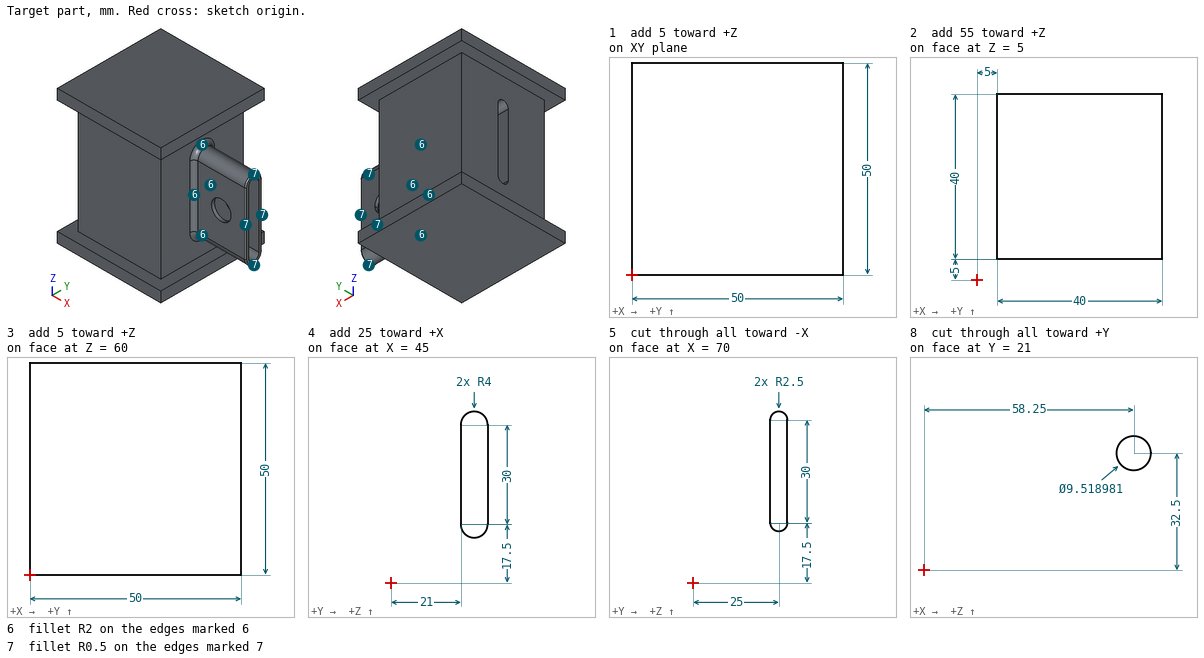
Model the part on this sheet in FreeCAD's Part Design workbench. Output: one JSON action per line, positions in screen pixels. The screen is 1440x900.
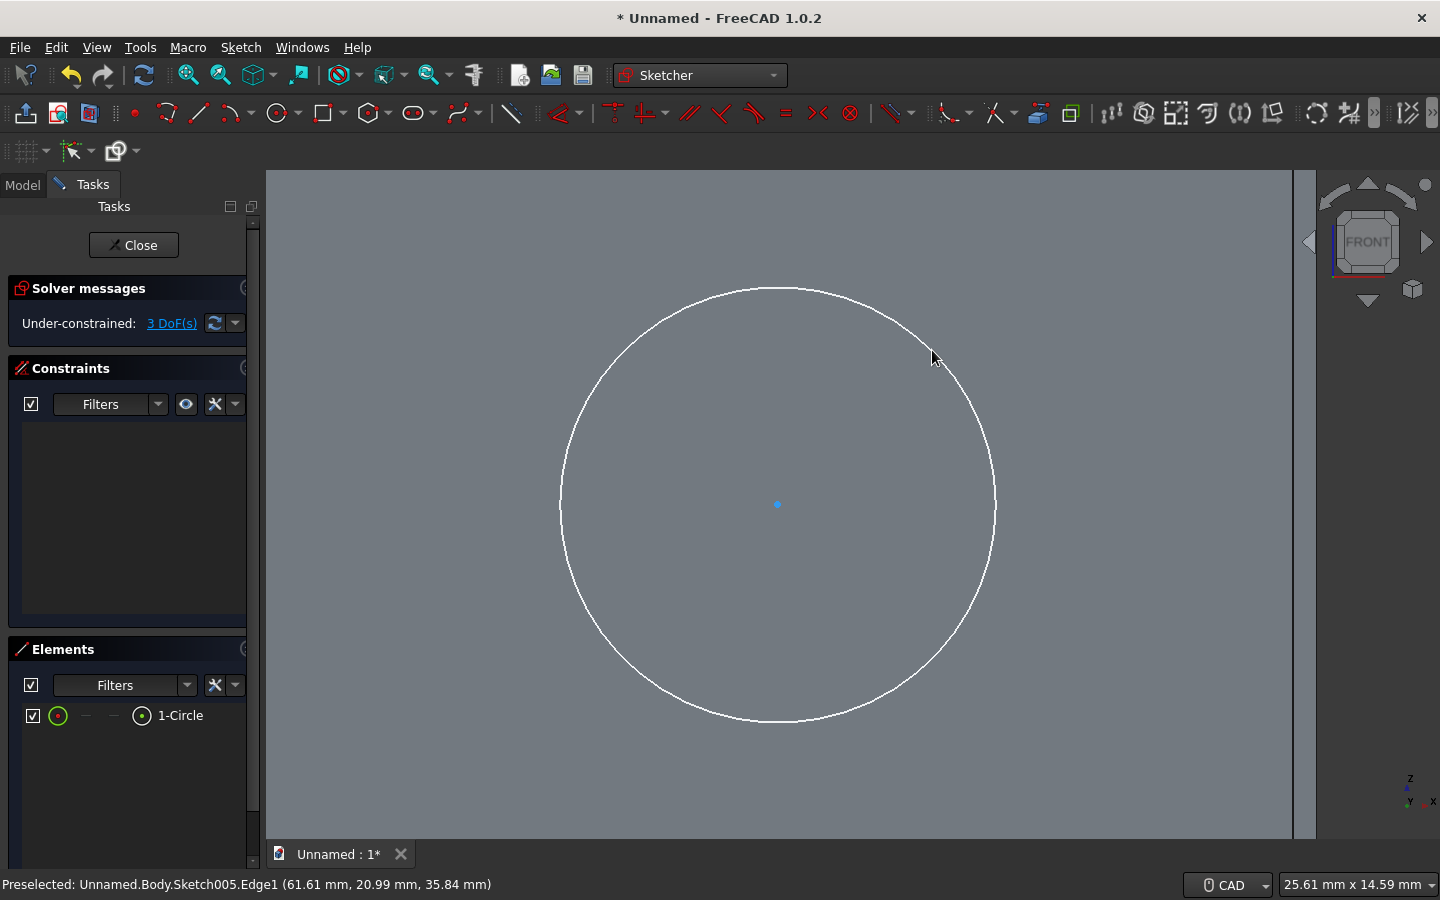
{"action": "left_click", "coordinate": [558, 114]}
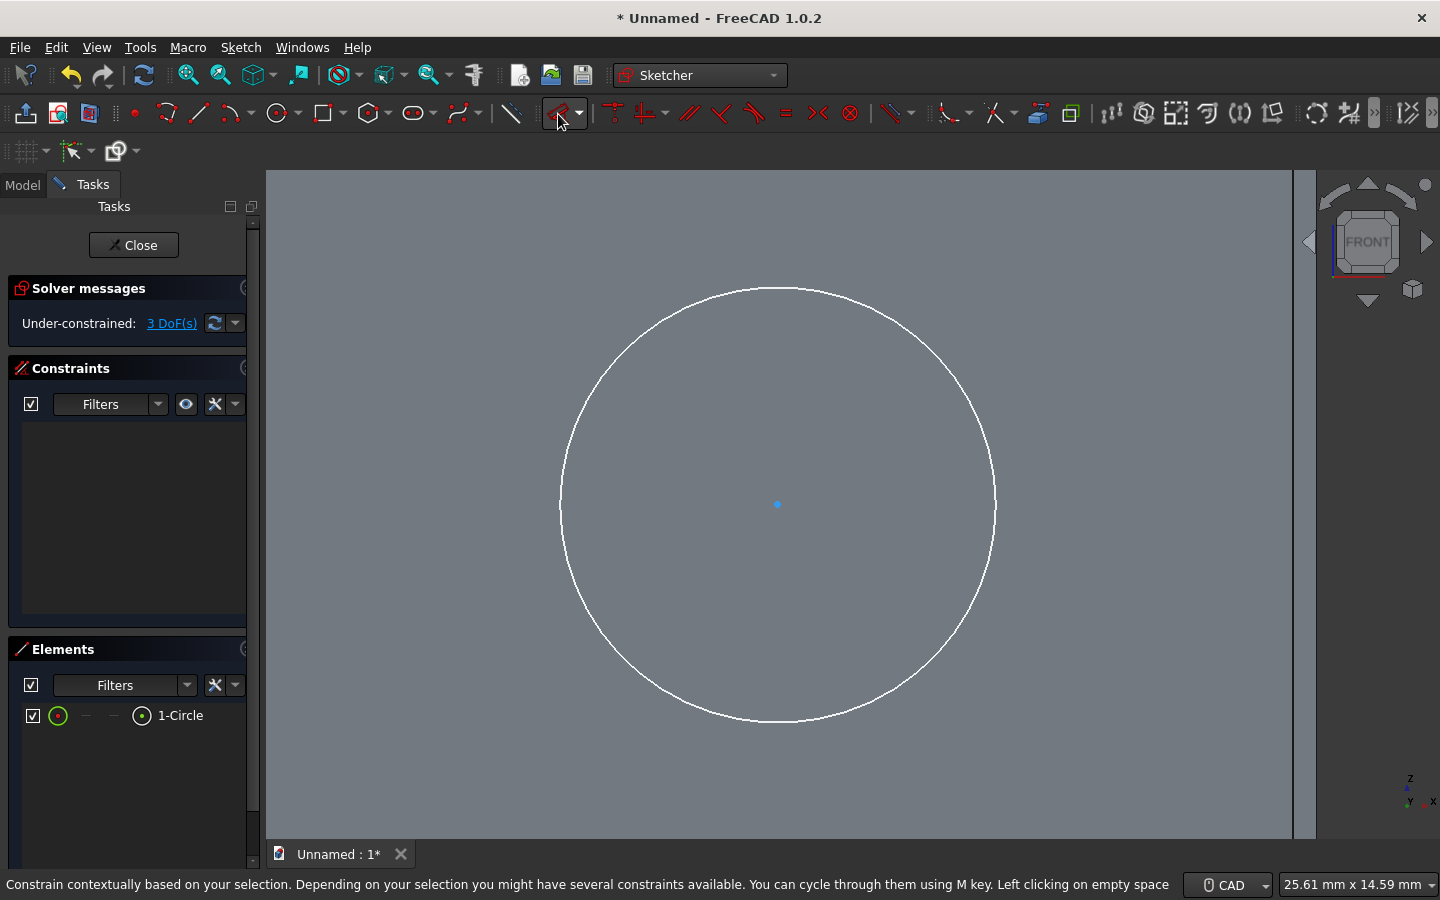
{"action": "left_click", "coordinate": [932, 351]}
{"action": "left_click", "coordinate": [955, 328]}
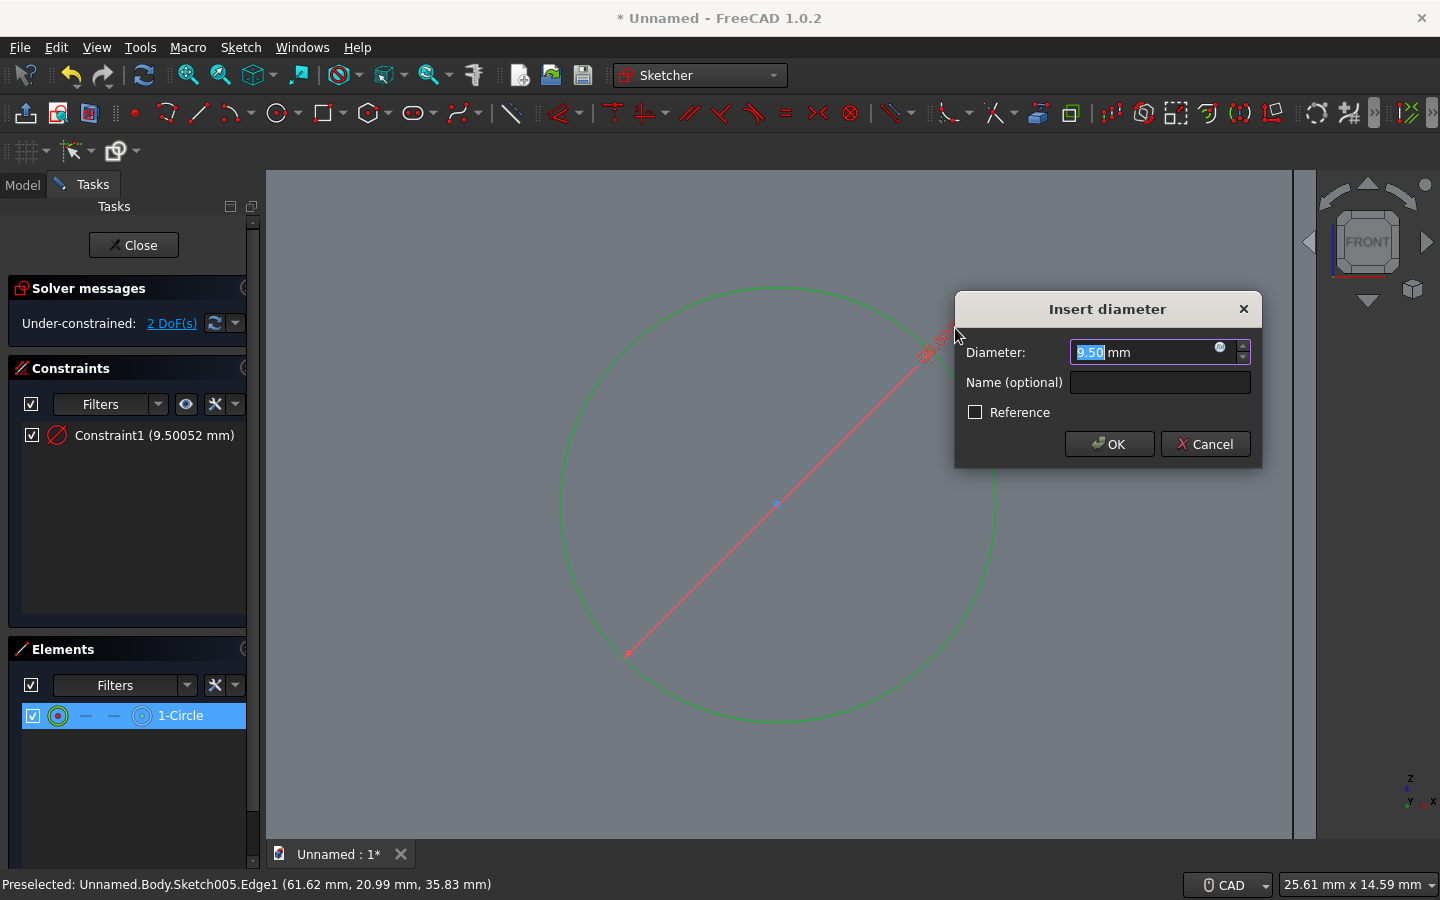
{"action": "type", "text": "9.518981"}
{"action": "key", "text": "Return"}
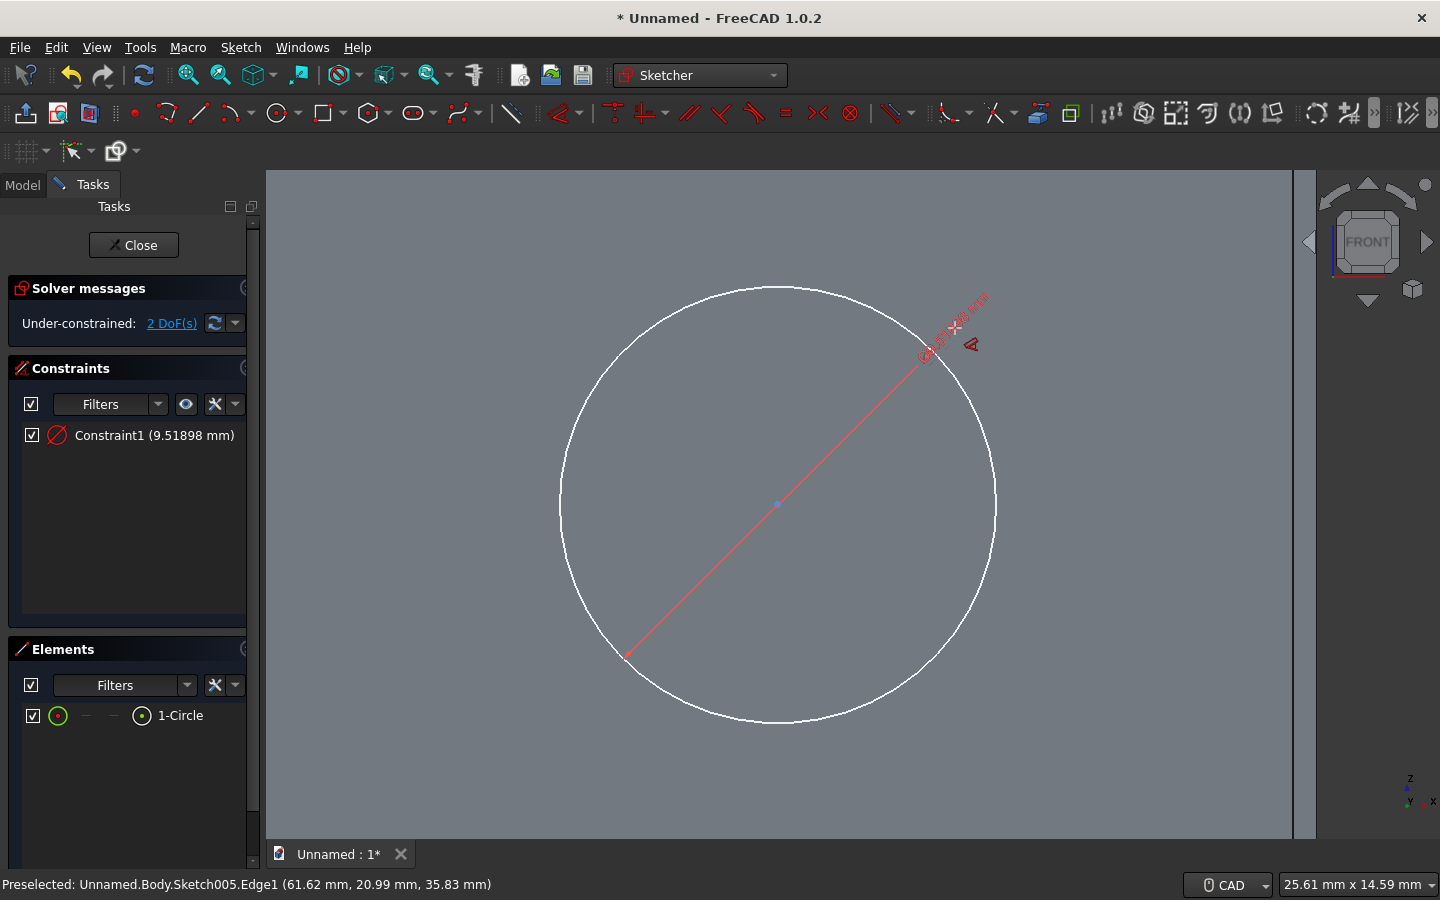
{"action": "left_click", "coordinate": [778, 505]}
{"action": "left_click", "coordinate": [812, 658]}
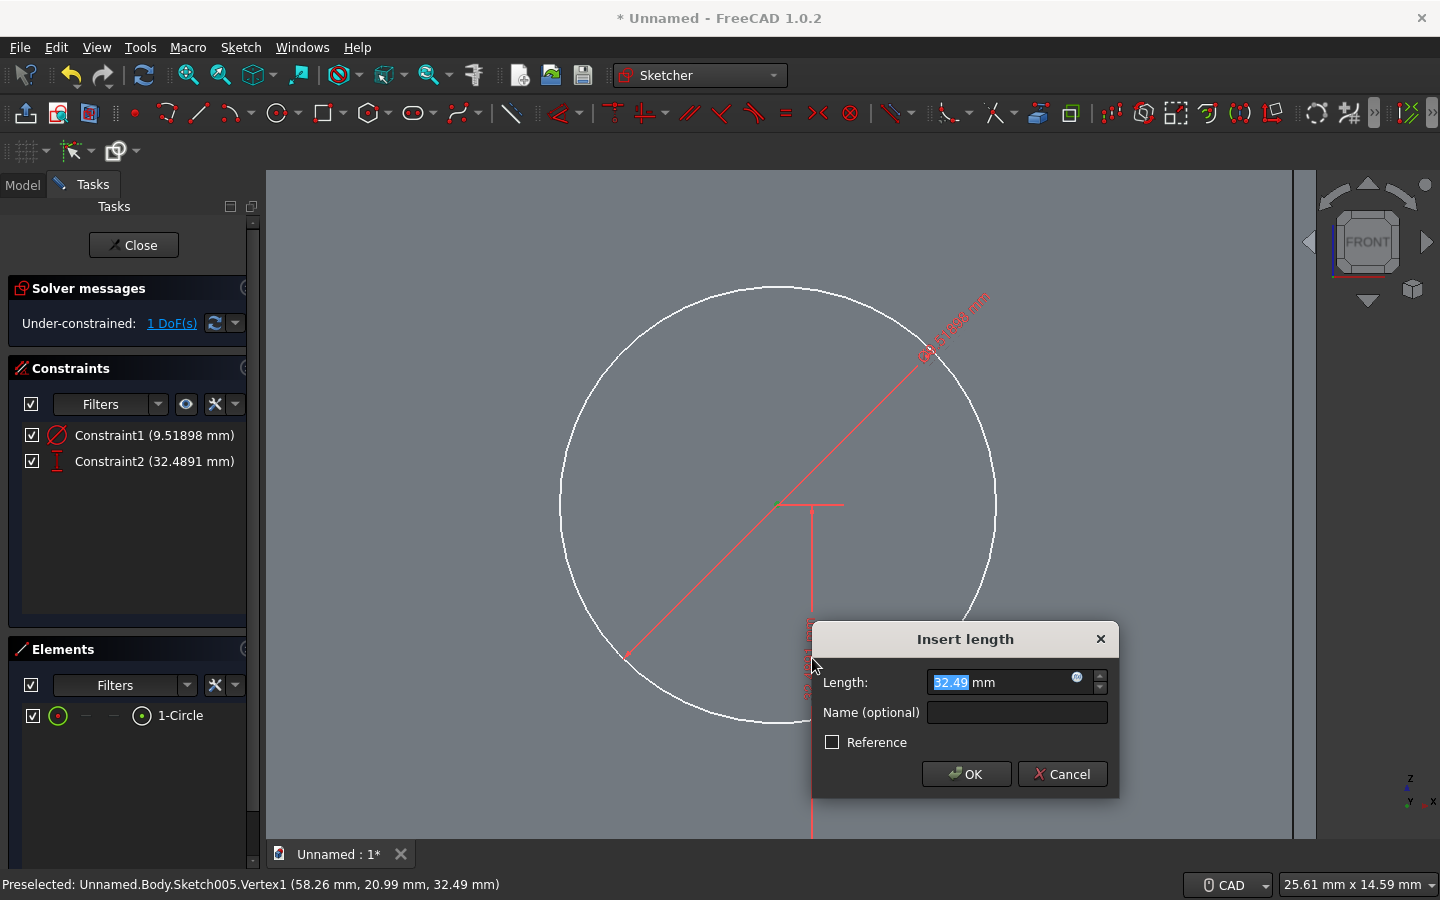
{"action": "type", "text": "32.5"}
{"action": "key", "text": "Return"}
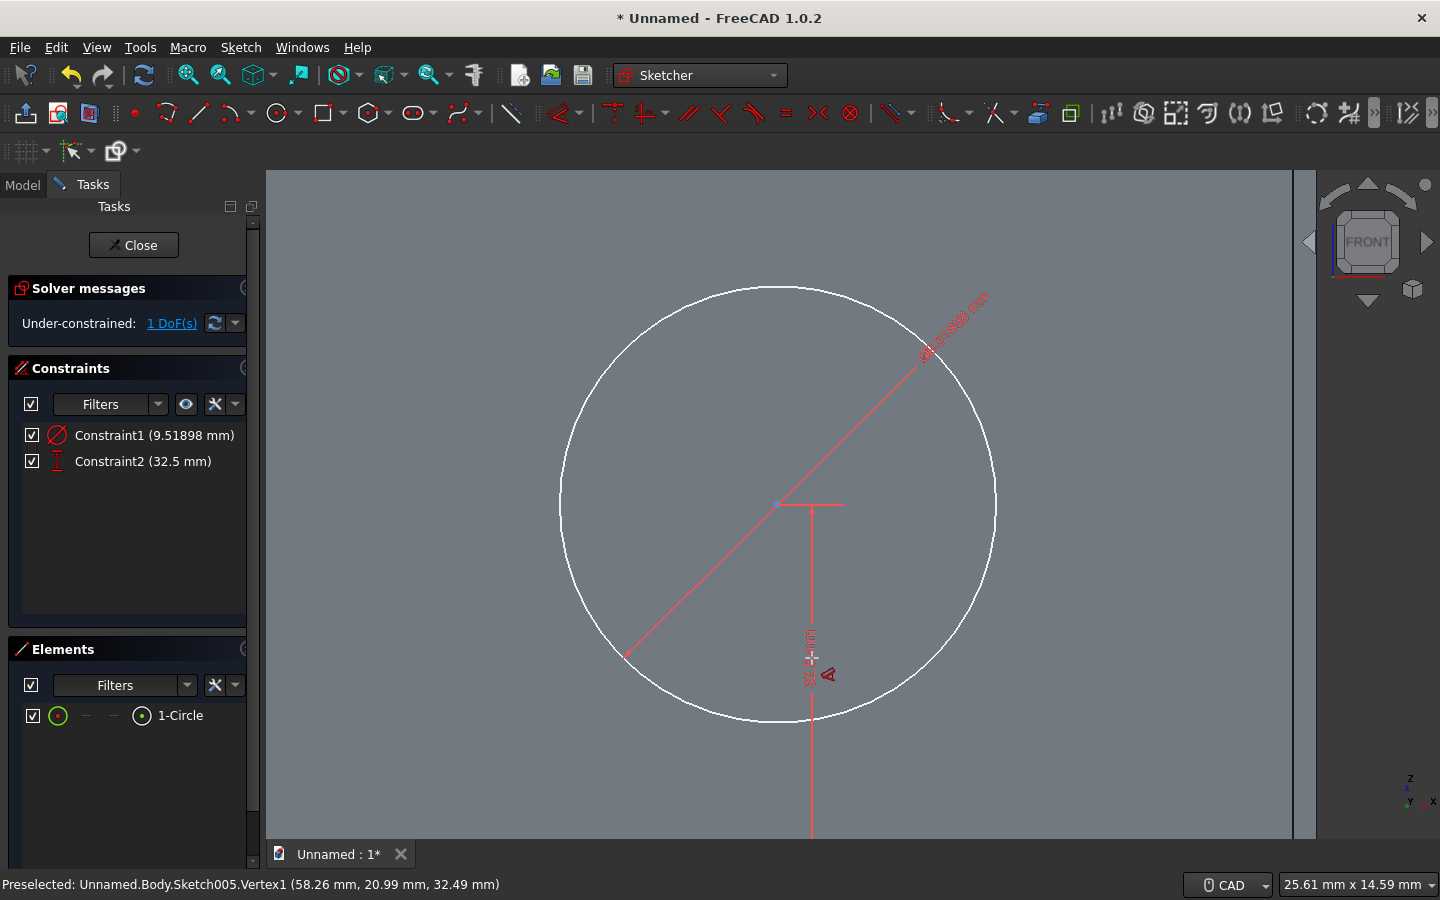
{"action": "left_click", "coordinate": [778, 504]}
{"action": "left_click", "coordinate": [536, 470]}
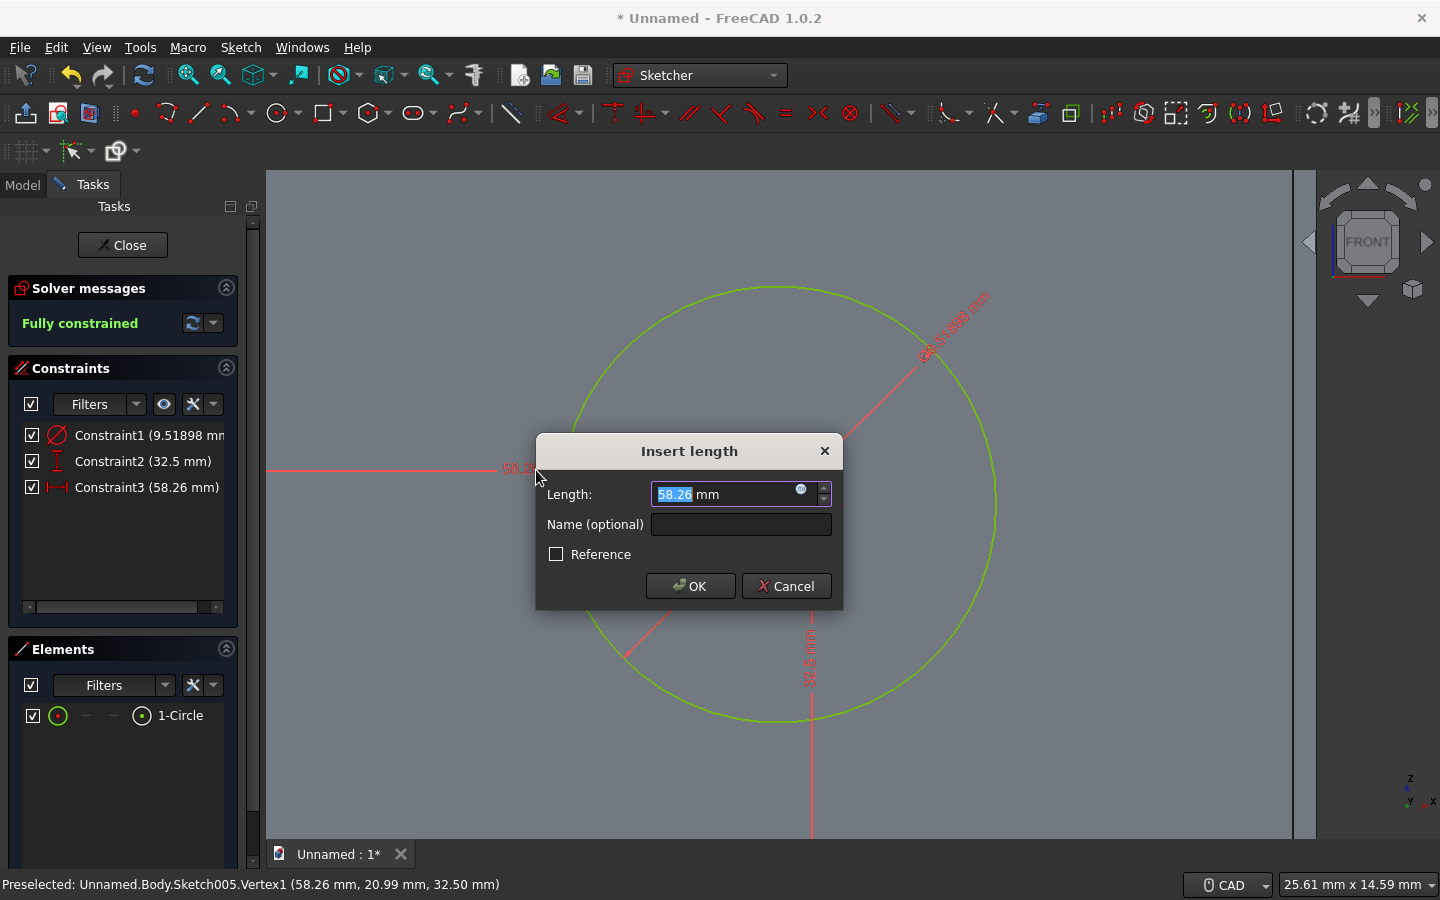
{"action": "type", "text": "58.25"}
{"action": "key", "text": "Return"}
{"action": "key", "text": "Escape"}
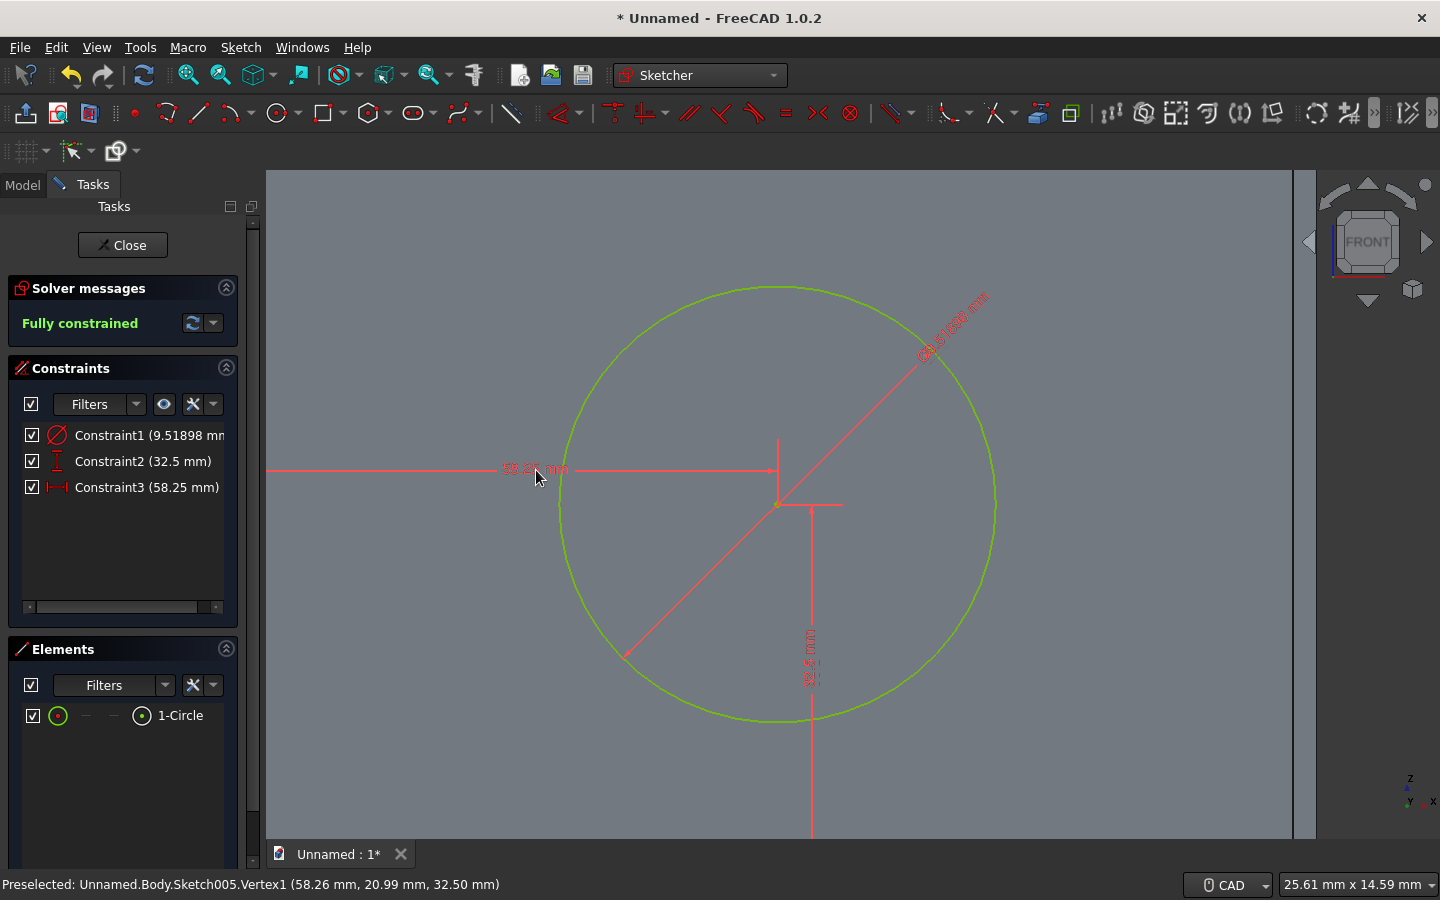
{"action": "left_click", "coordinate": [123, 245]}